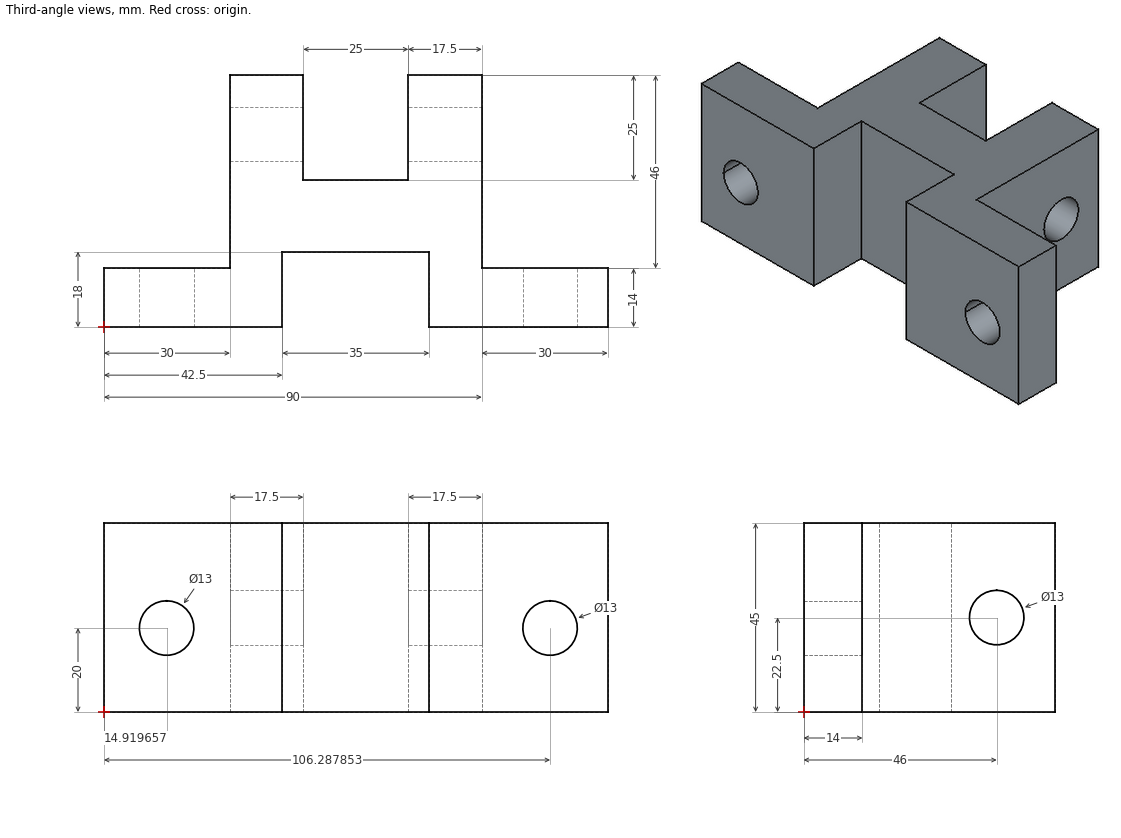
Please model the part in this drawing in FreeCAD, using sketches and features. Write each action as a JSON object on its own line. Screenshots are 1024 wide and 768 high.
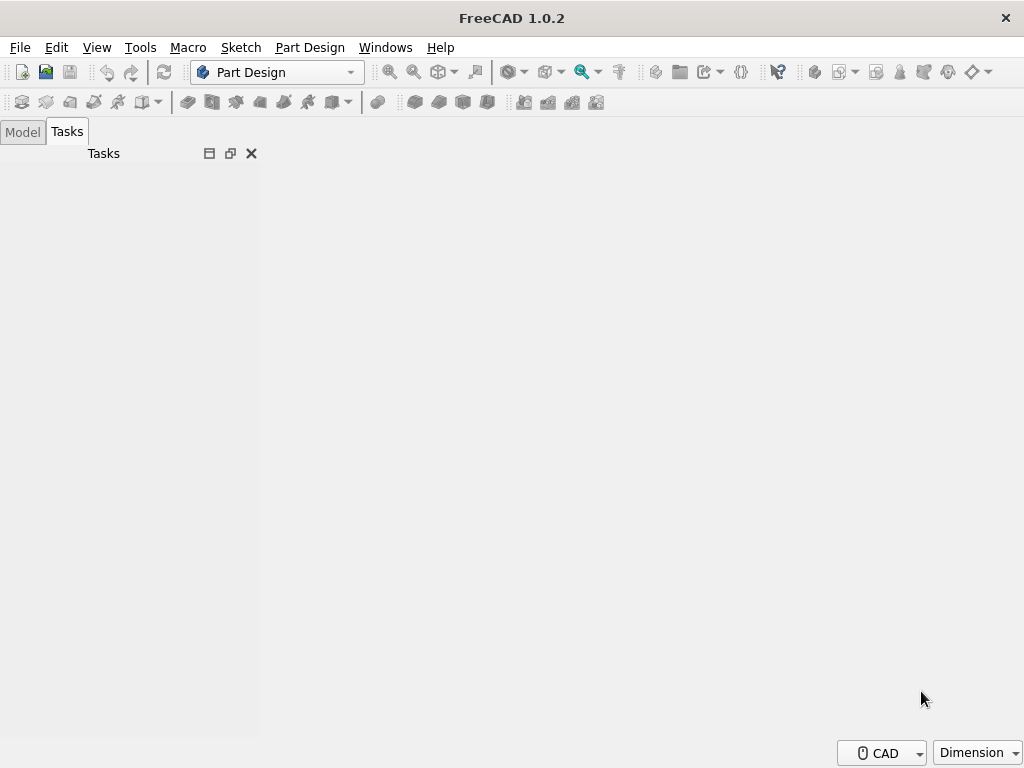
{"action": "left_click", "coordinate": [22, 72]}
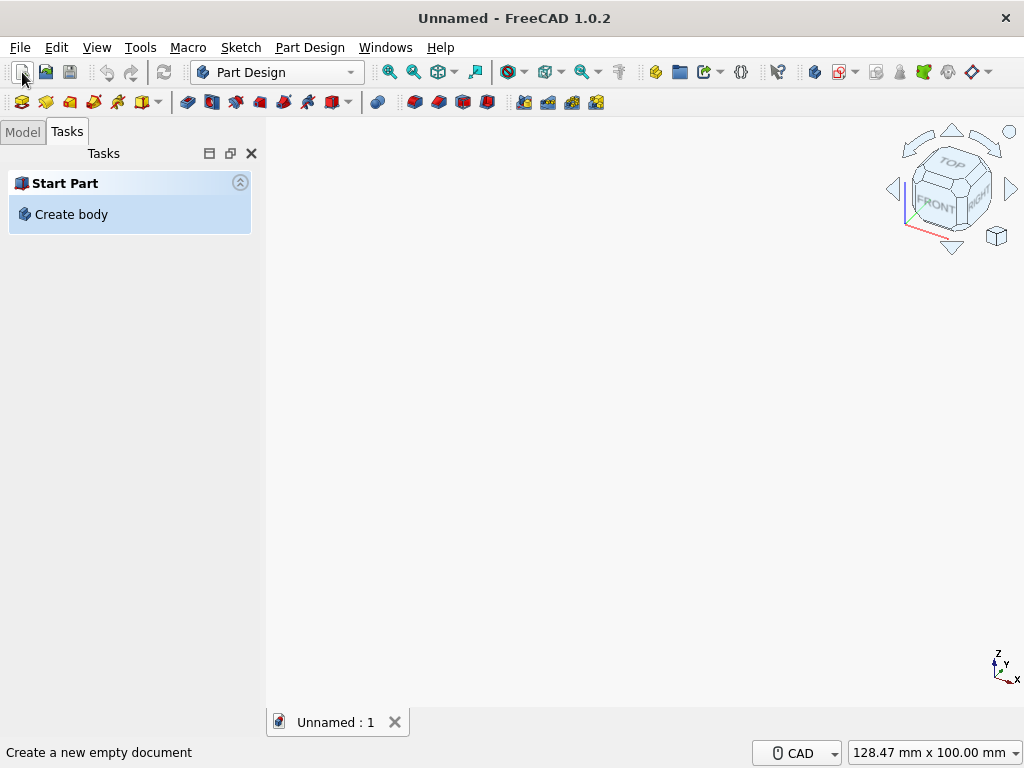
{"action": "left_click", "coordinate": [840, 72]}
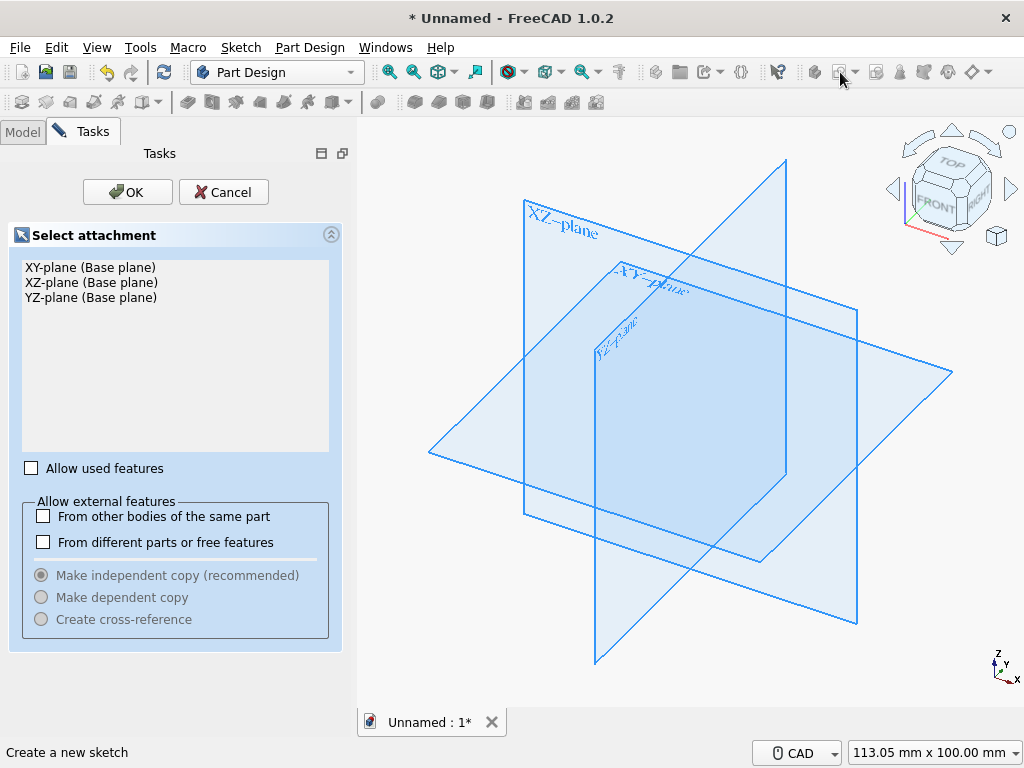
{"action": "left_click", "coordinate": [82, 268]}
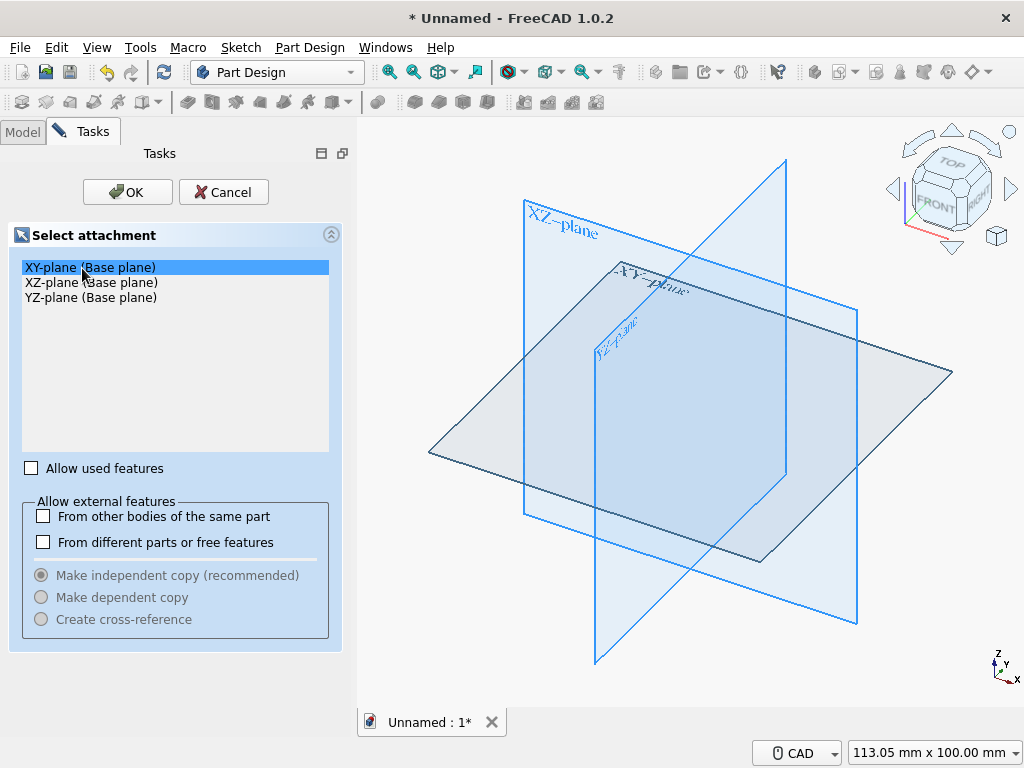
{"action": "left_click", "coordinate": [128, 192]}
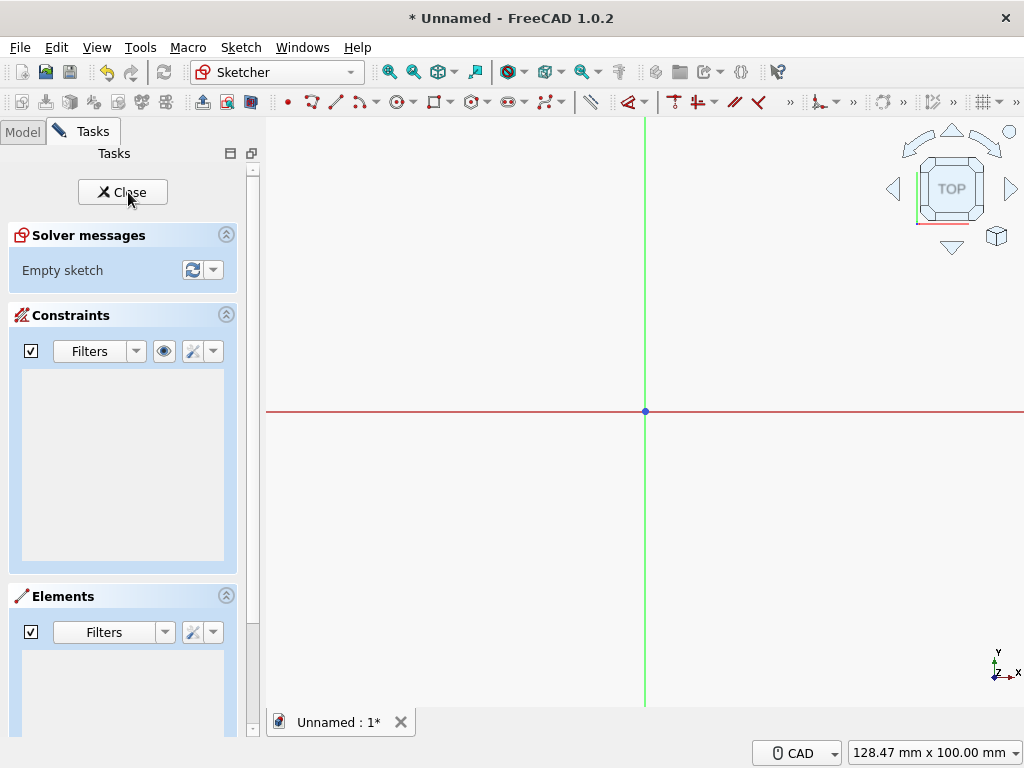
{"action": "scroll", "coordinate": [294, 556], "scroll_direction": "down", "scroll_amount": 4}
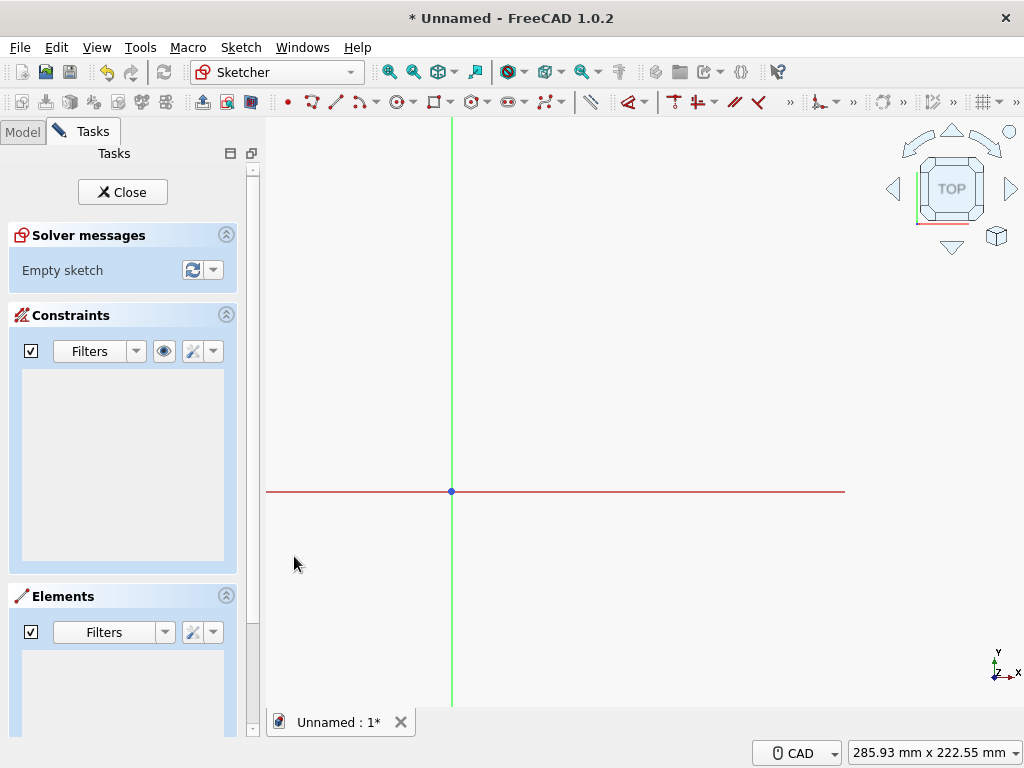
{"action": "left_click", "coordinate": [312, 102]}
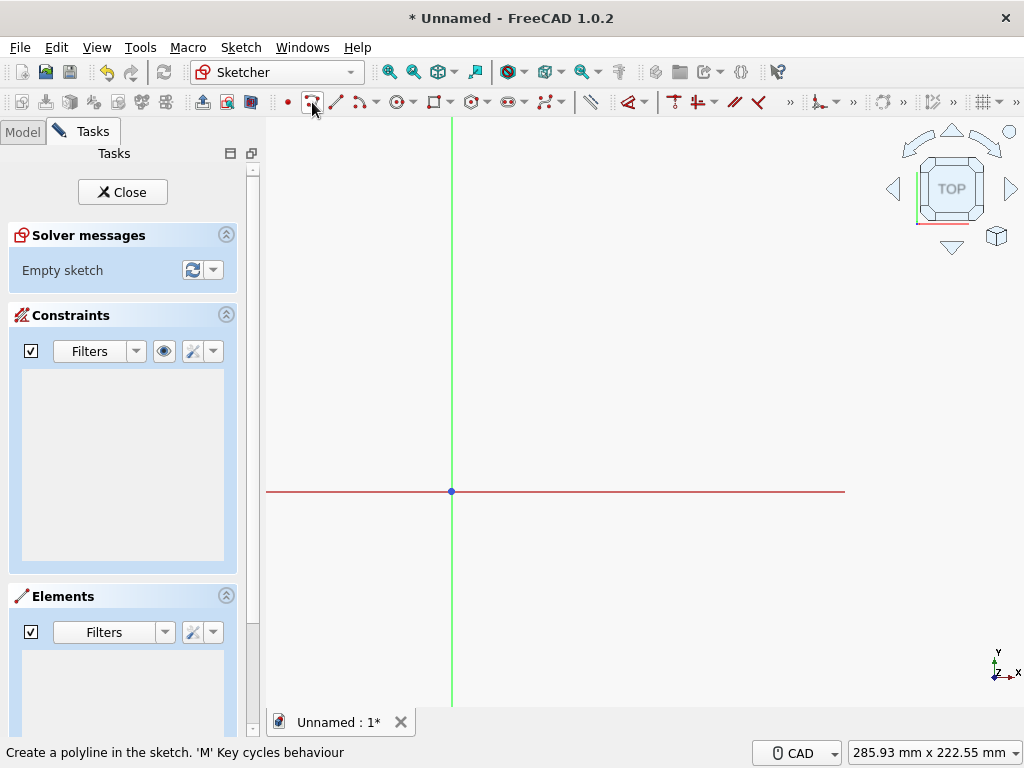
{"action": "left_click", "coordinate": [452, 492]}
{"action": "left_click", "coordinate": [564, 483]}
{"action": "left_click", "coordinate": [564, 444]}
{"action": "left_click", "coordinate": [657, 444]}
{"action": "left_click", "coordinate": [657, 492]}
{"action": "left_click", "coordinate": [770, 483]}
{"action": "left_click", "coordinate": [770, 455]}
{"action": "left_click", "coordinate": [690, 455]}
{"action": "left_click", "coordinate": [690, 333]}
{"action": "left_click", "coordinate": [644, 333]}
{"action": "left_click", "coordinate": [644, 399]}
{"action": "left_click", "coordinate": [578, 399]}
{"action": "left_click", "coordinate": [578, 333]}
{"action": "left_click", "coordinate": [531, 333]}
{"action": "left_click", "coordinate": [531, 455]}
{"action": "left_click", "coordinate": [461, 455]}
{"action": "left_click", "coordinate": [452, 492]}
{"action": "key", "text": "Escape"}
{"action": "key", "text": "Escape"}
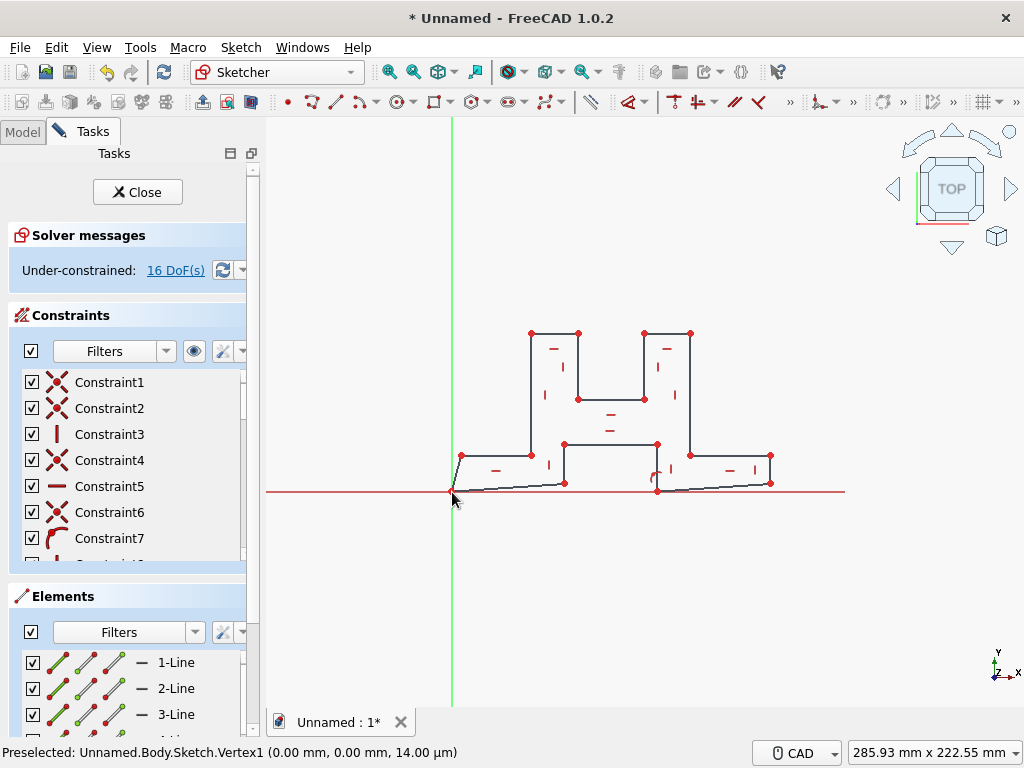
{"action": "left_click", "coordinate": [485, 489]}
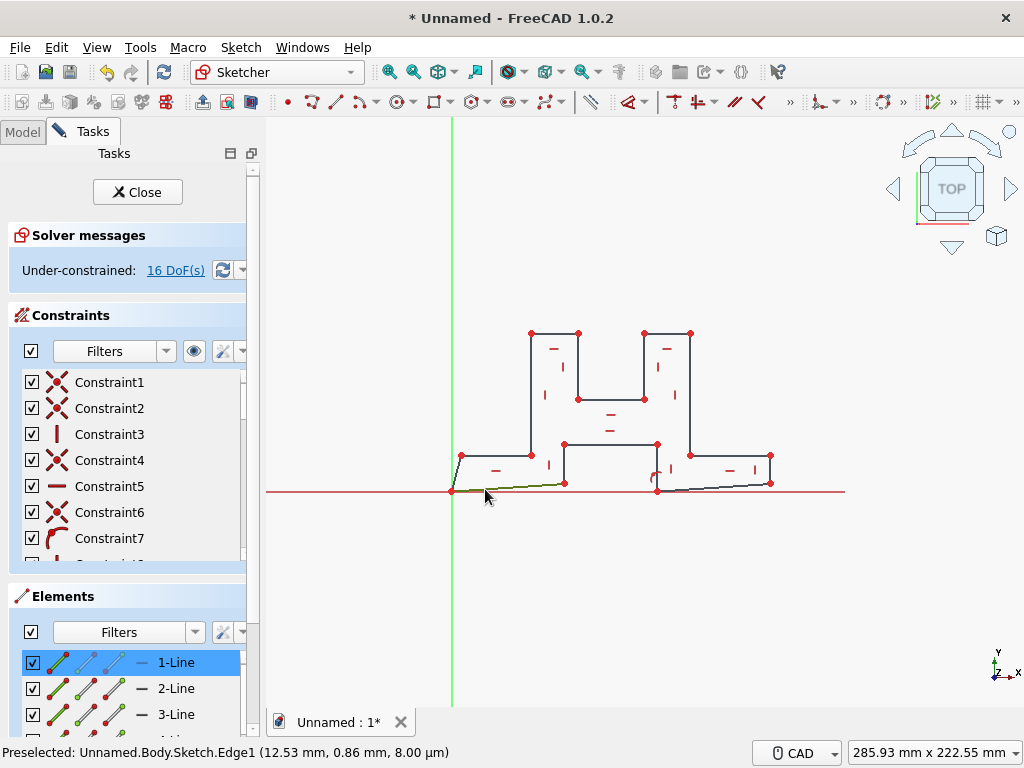
{"action": "key", "text": "h"}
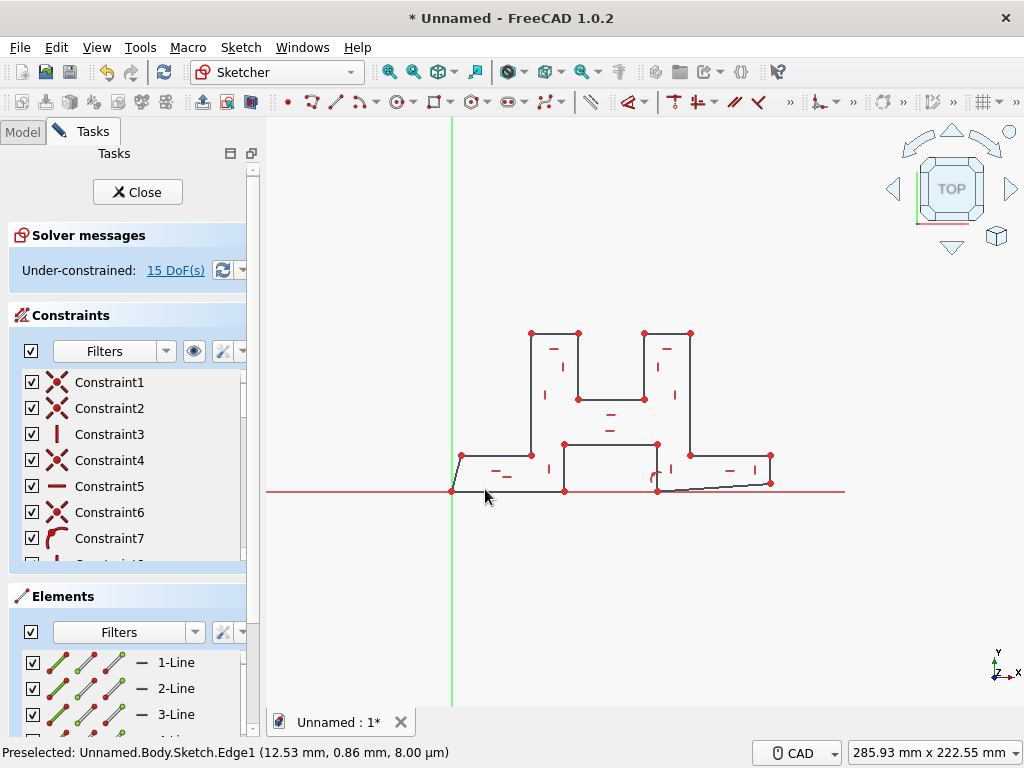
{"action": "left_click", "coordinate": [691, 489]}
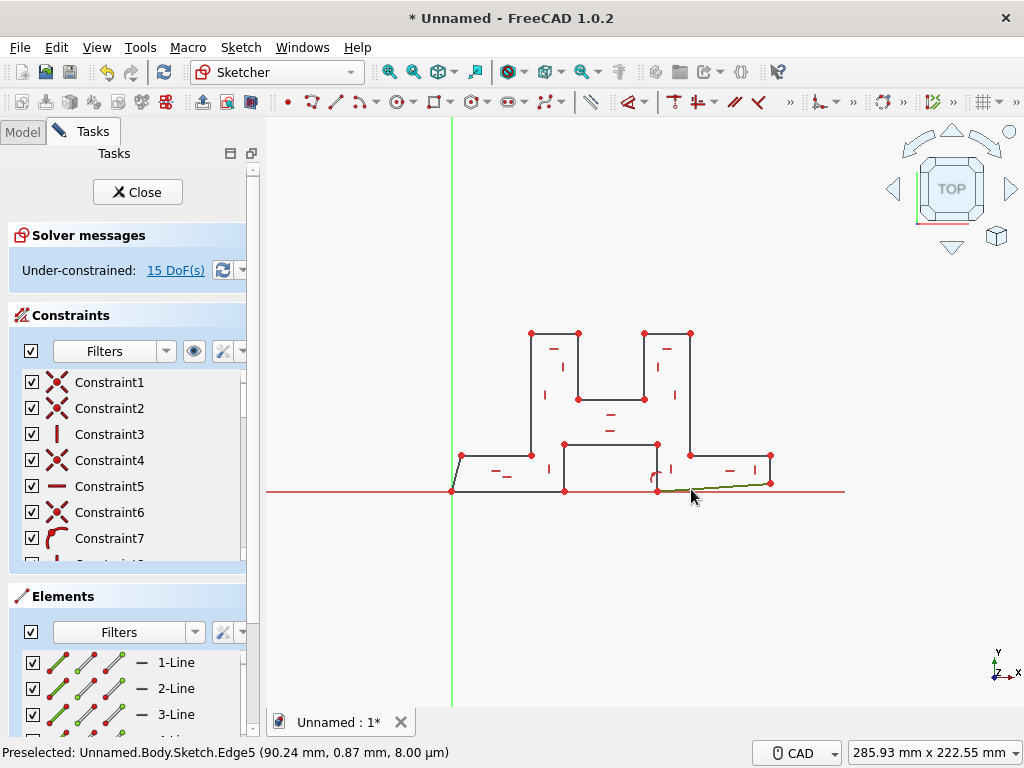
{"action": "key", "text": "h"}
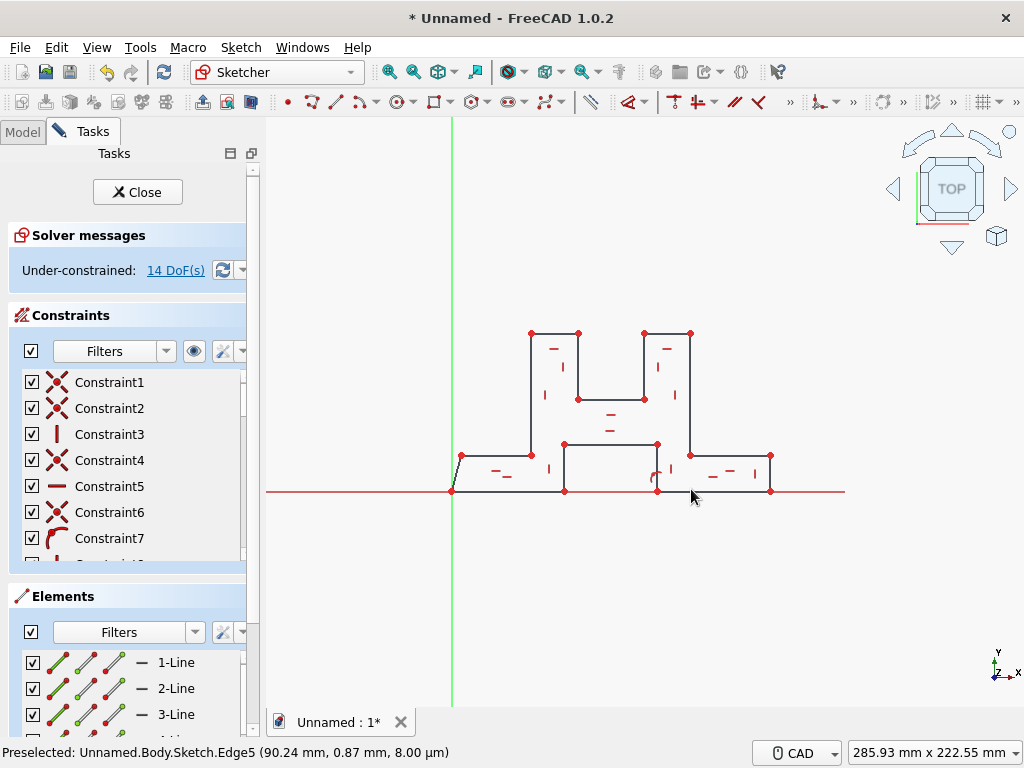
{"action": "scroll", "coordinate": [455, 481], "scroll_direction": "up", "scroll_amount": 2}